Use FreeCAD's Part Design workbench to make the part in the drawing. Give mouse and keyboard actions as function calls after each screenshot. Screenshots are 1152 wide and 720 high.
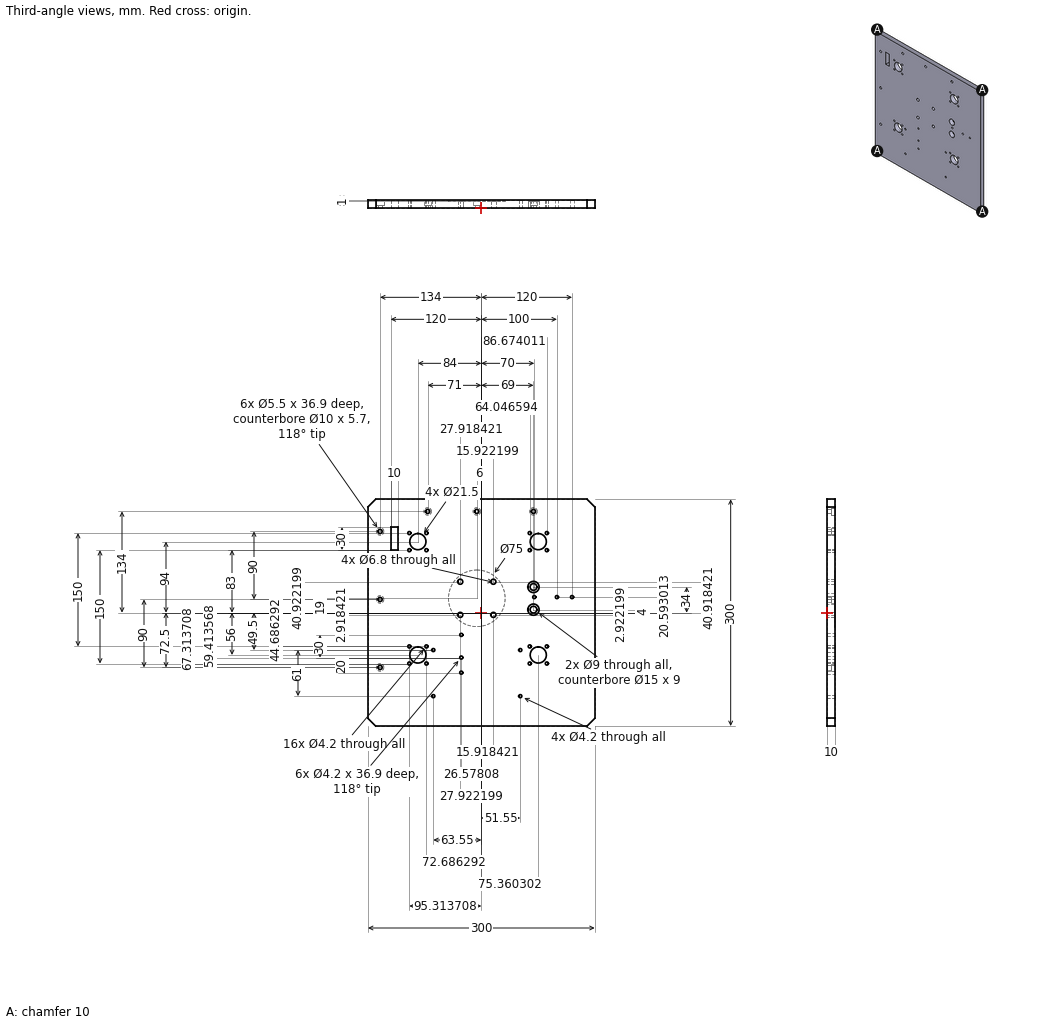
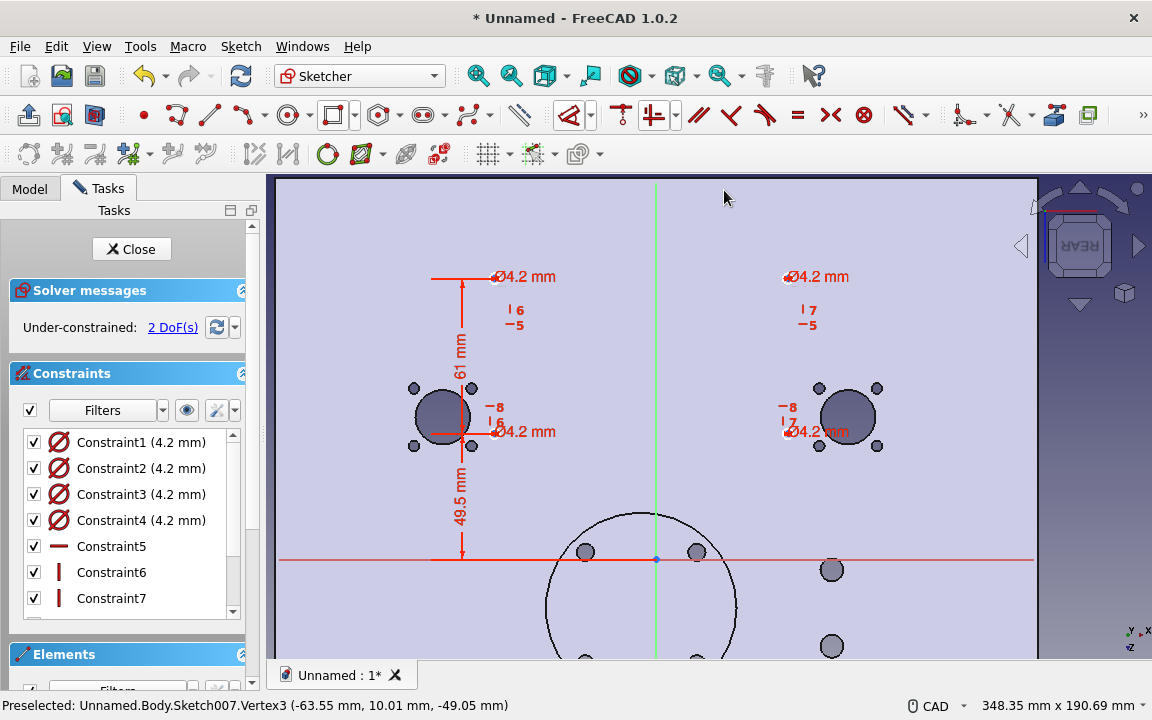
click(788, 279)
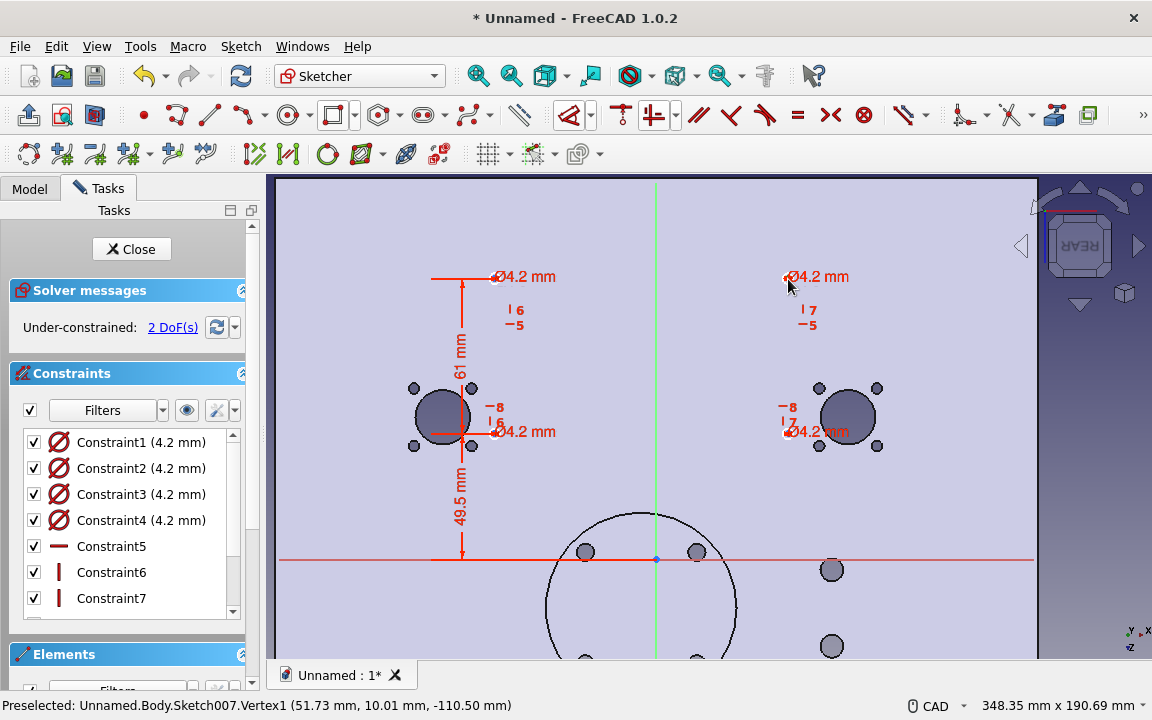
click(590, 116)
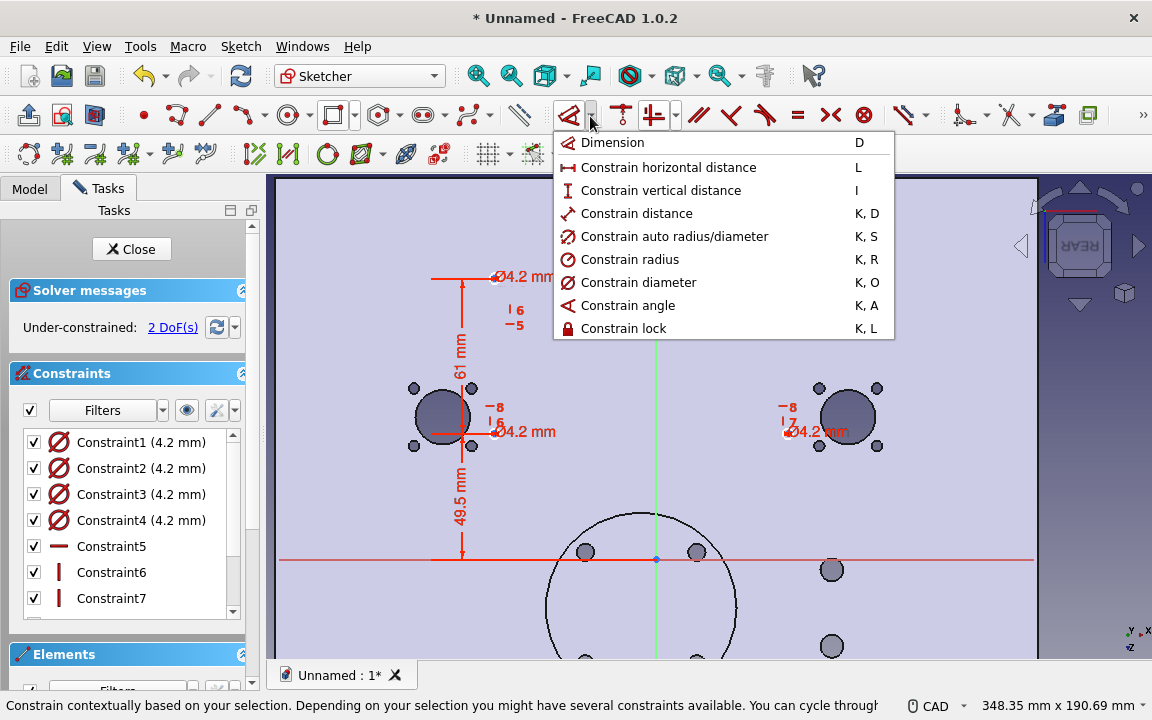
click(724, 168)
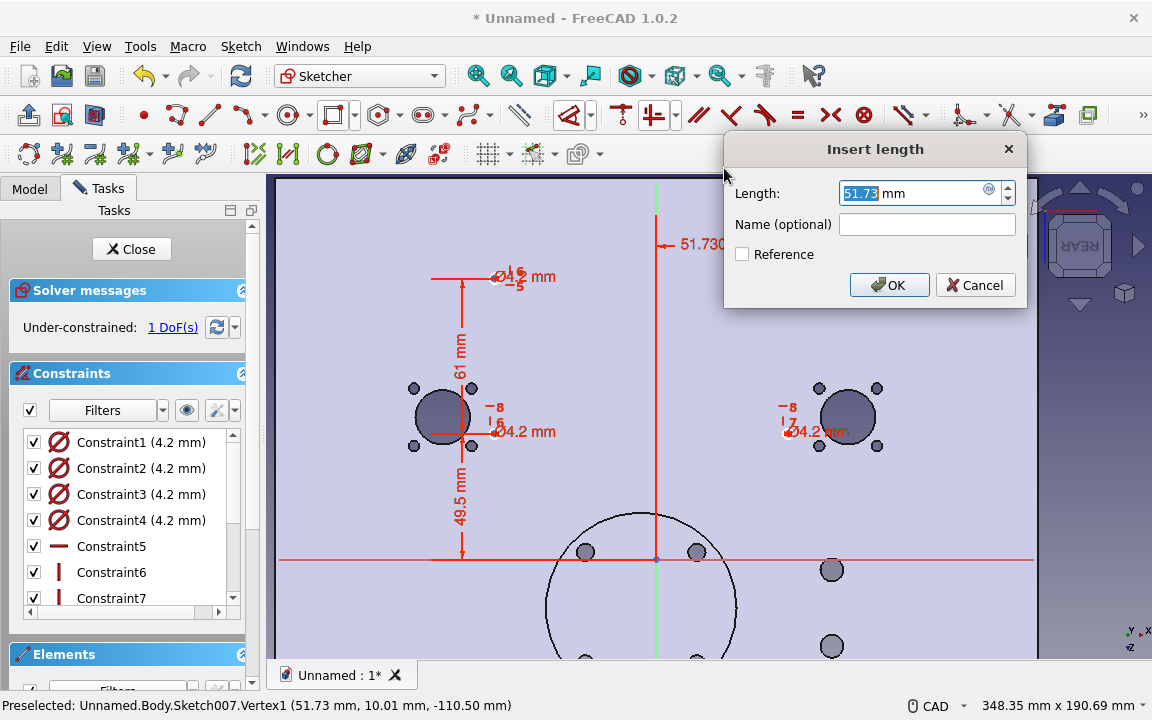
text(51.55)
key(Return)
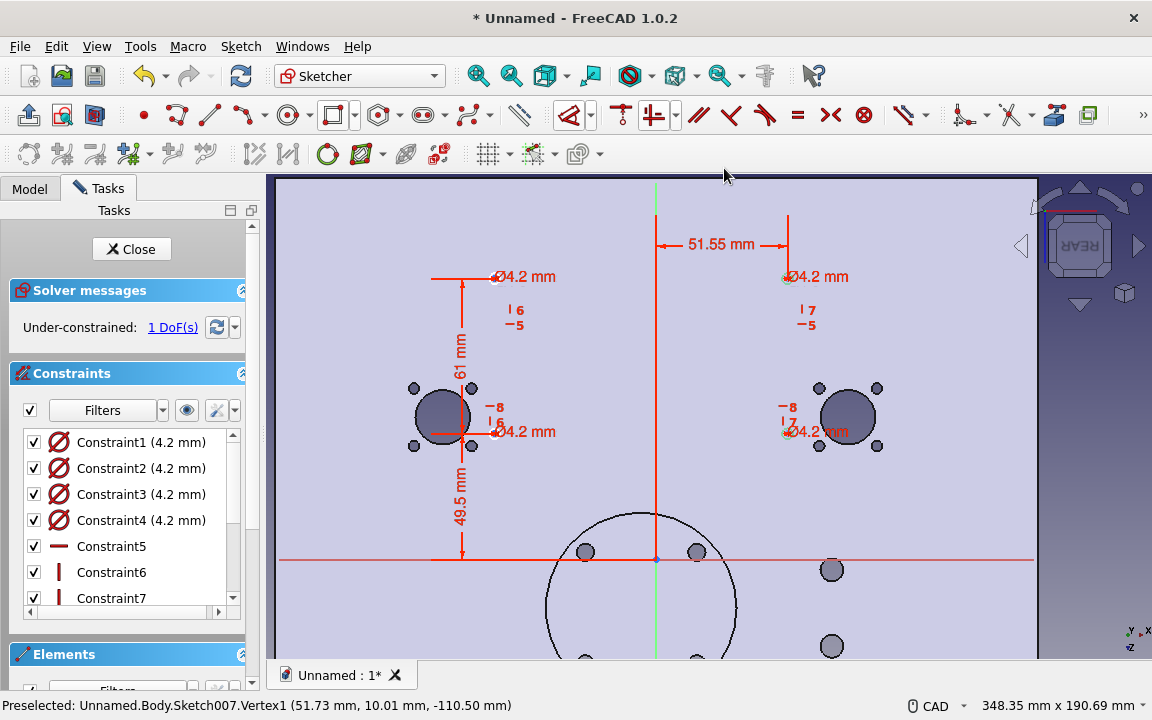
click(495, 279)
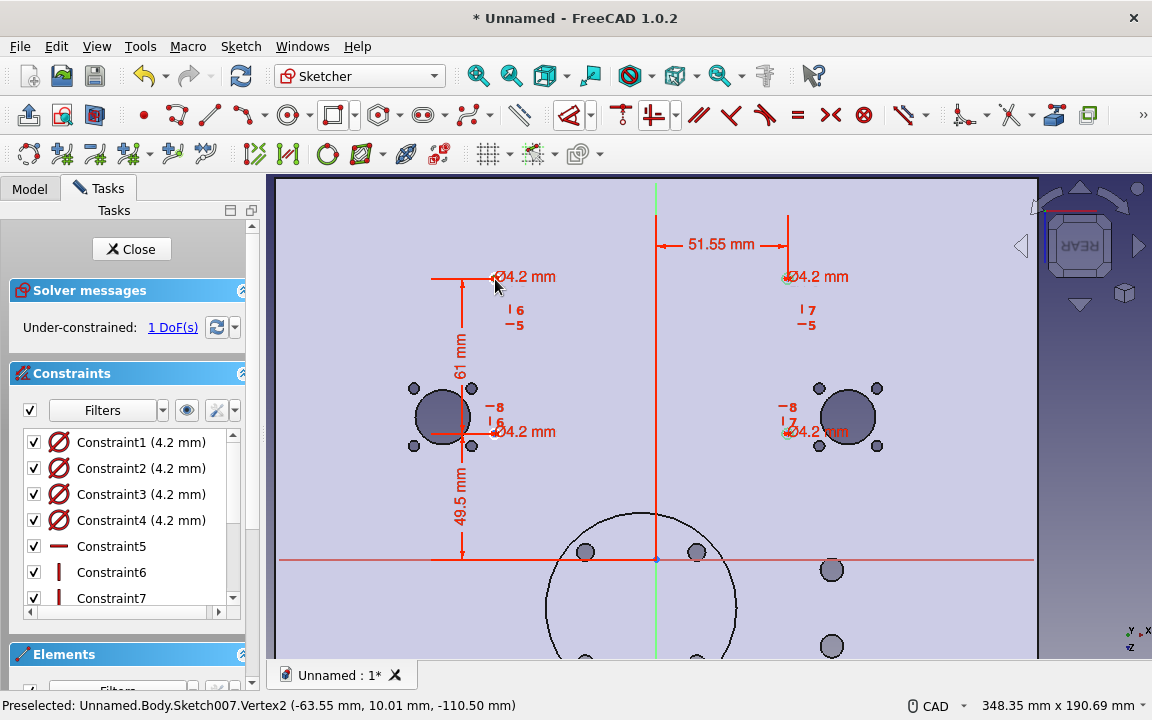
key(l)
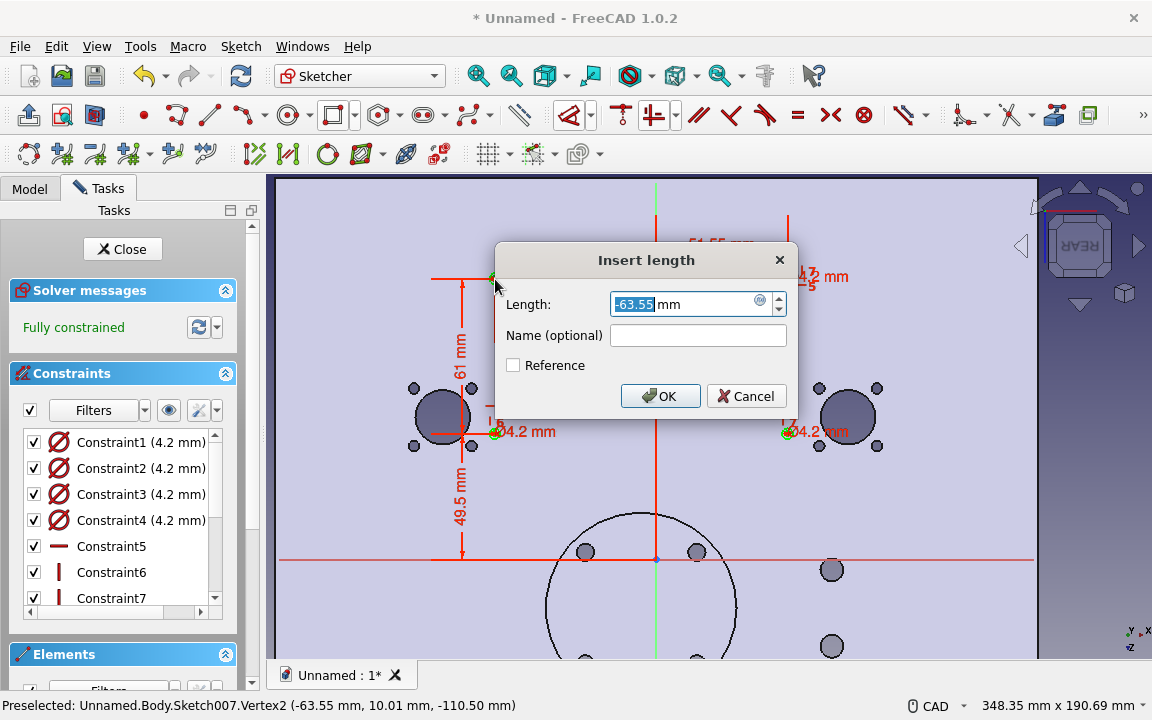
text(-63.55)
key(Return)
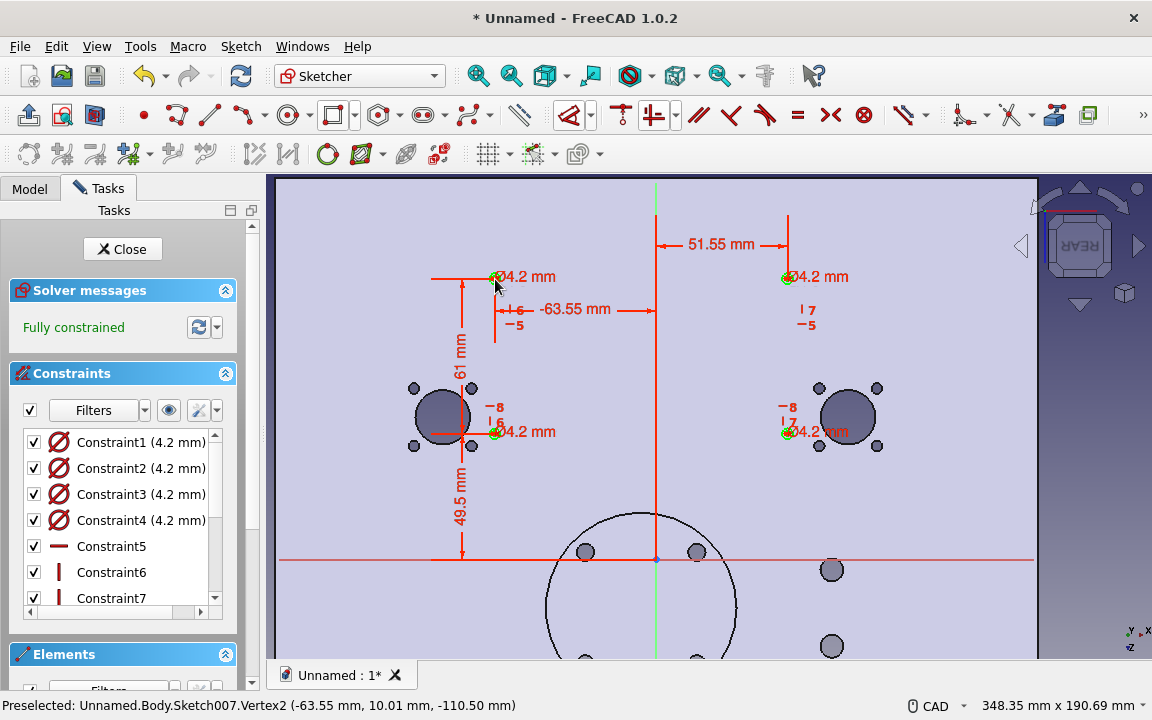
click(123, 249)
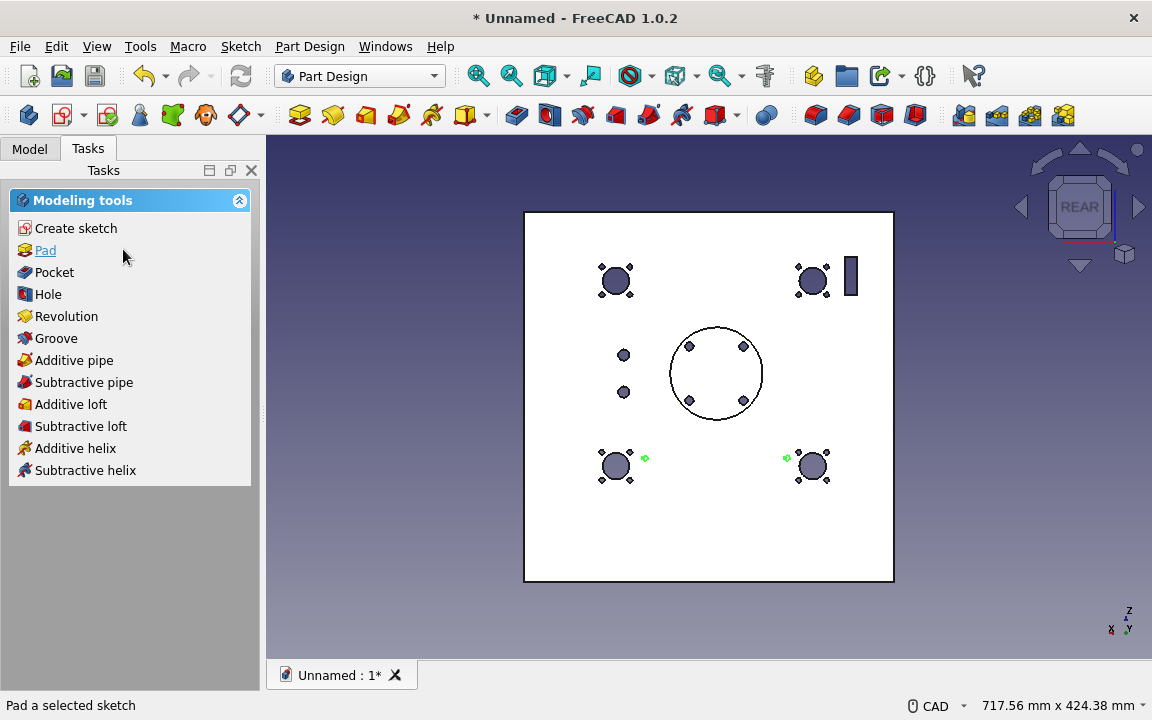
click(550, 116)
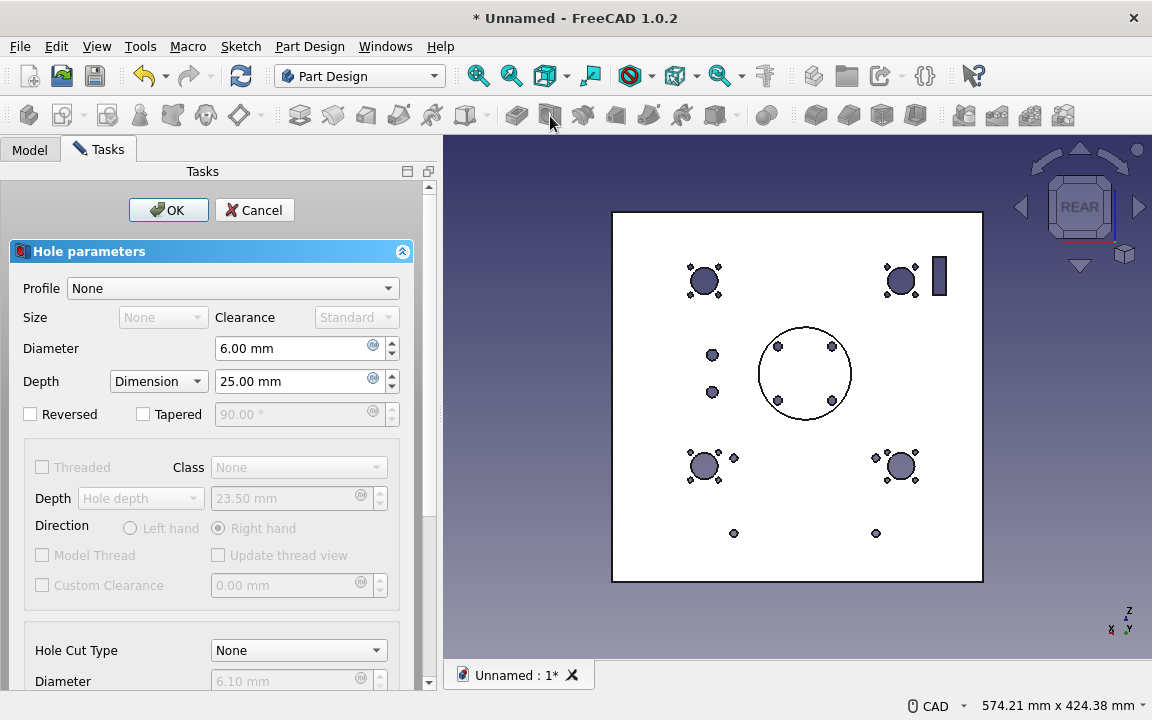
triple_click(300, 348)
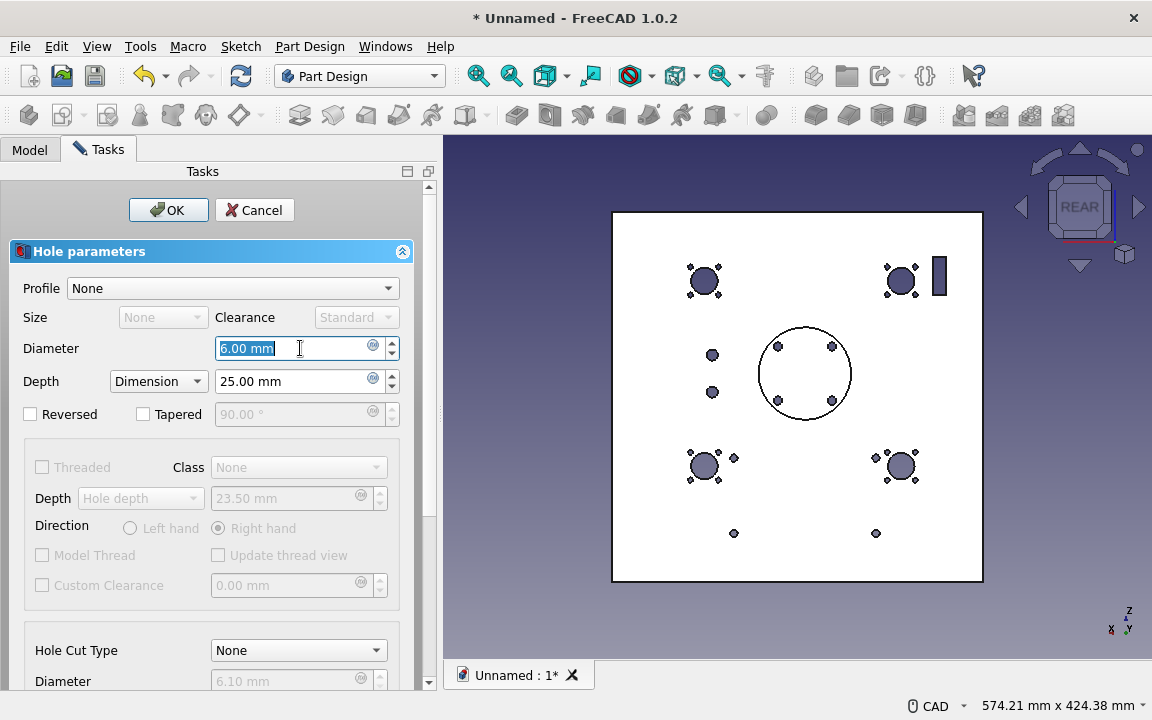
text(4.2)
key(Tab)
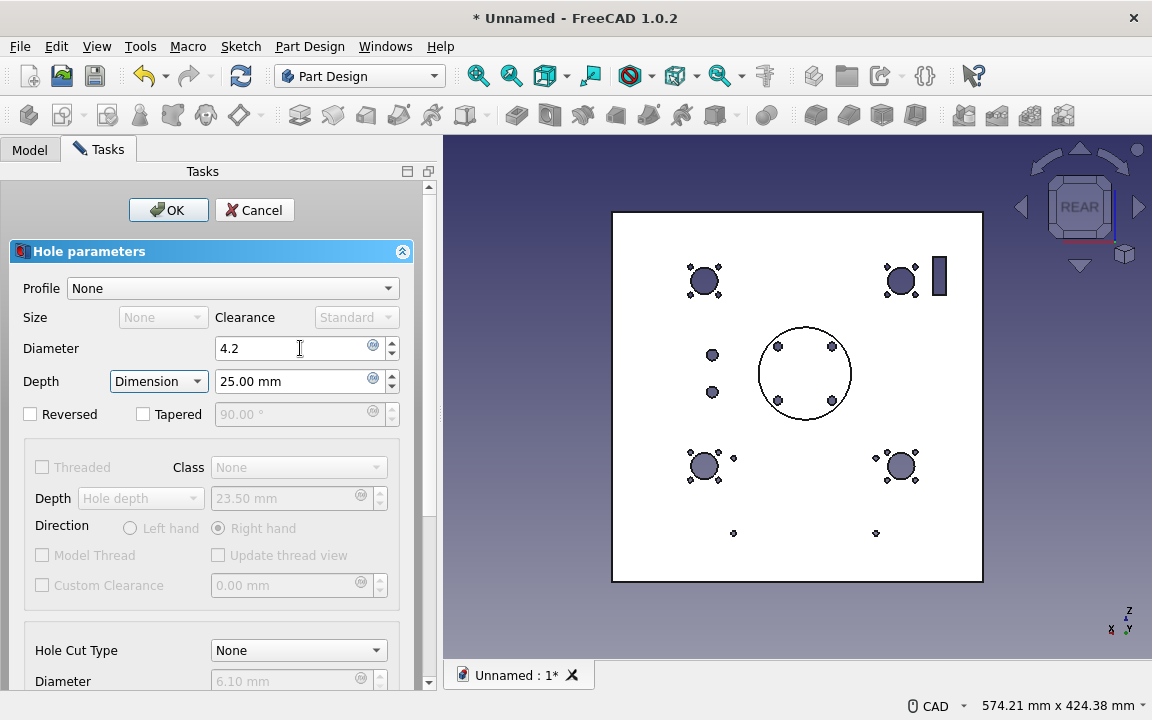
click(160, 382)